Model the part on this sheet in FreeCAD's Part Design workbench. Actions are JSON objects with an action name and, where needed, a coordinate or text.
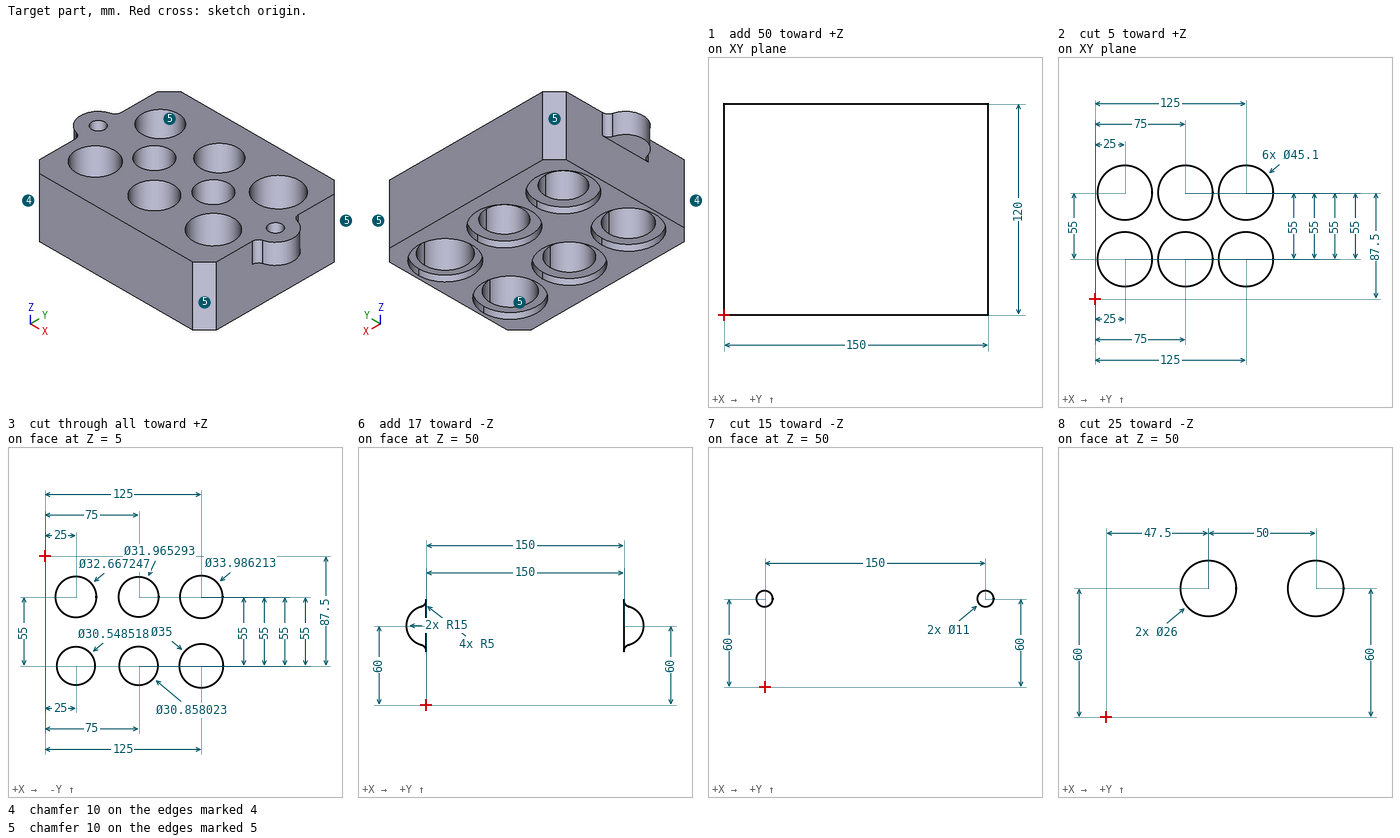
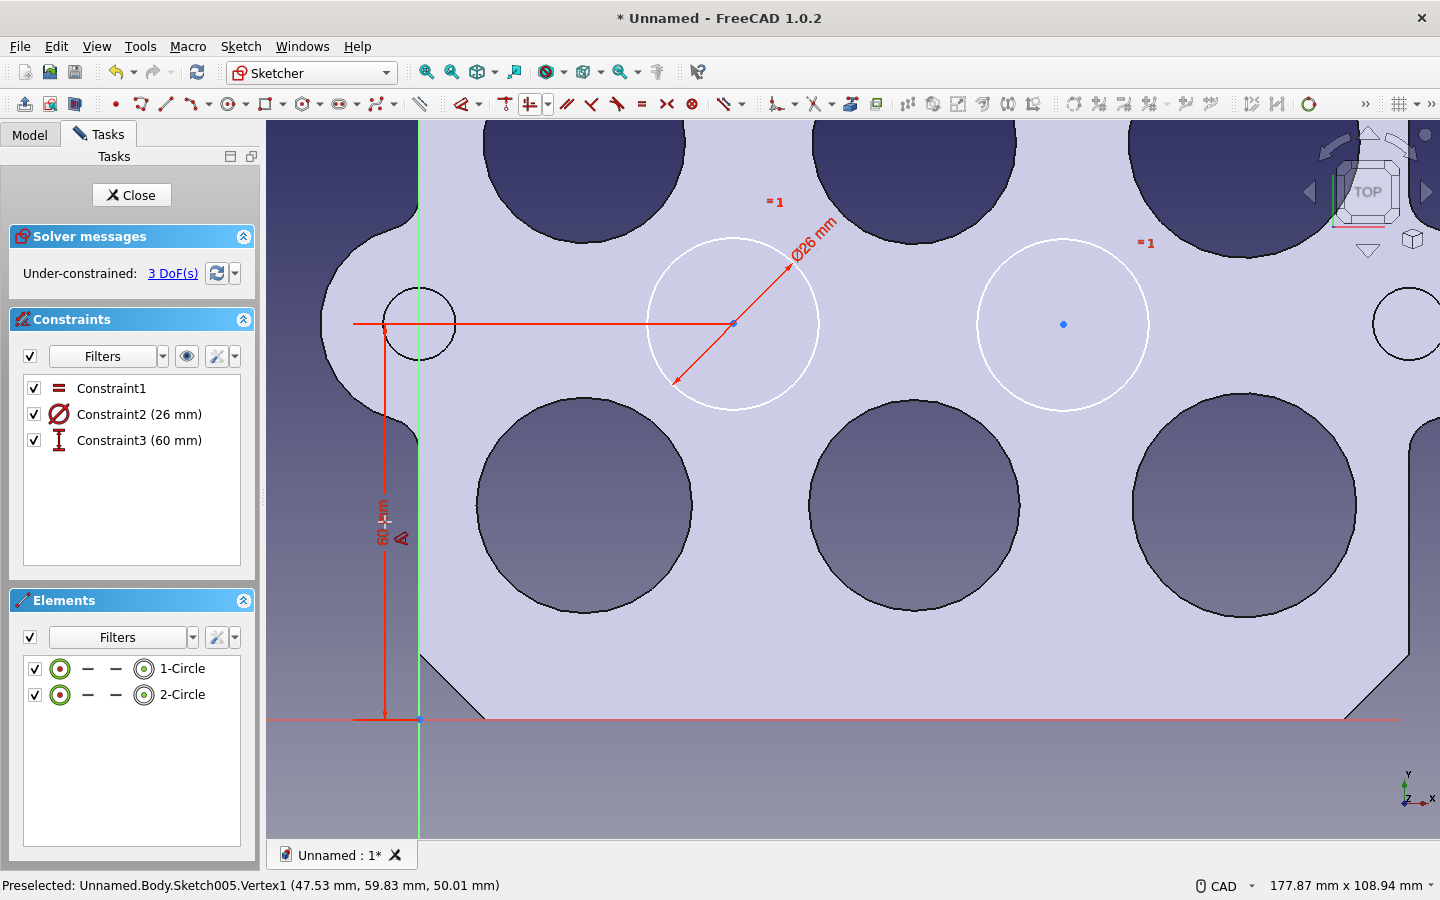
{"action": "left_click", "coordinate": [1063, 325]}
{"action": "left_click", "coordinate": [385, 432]}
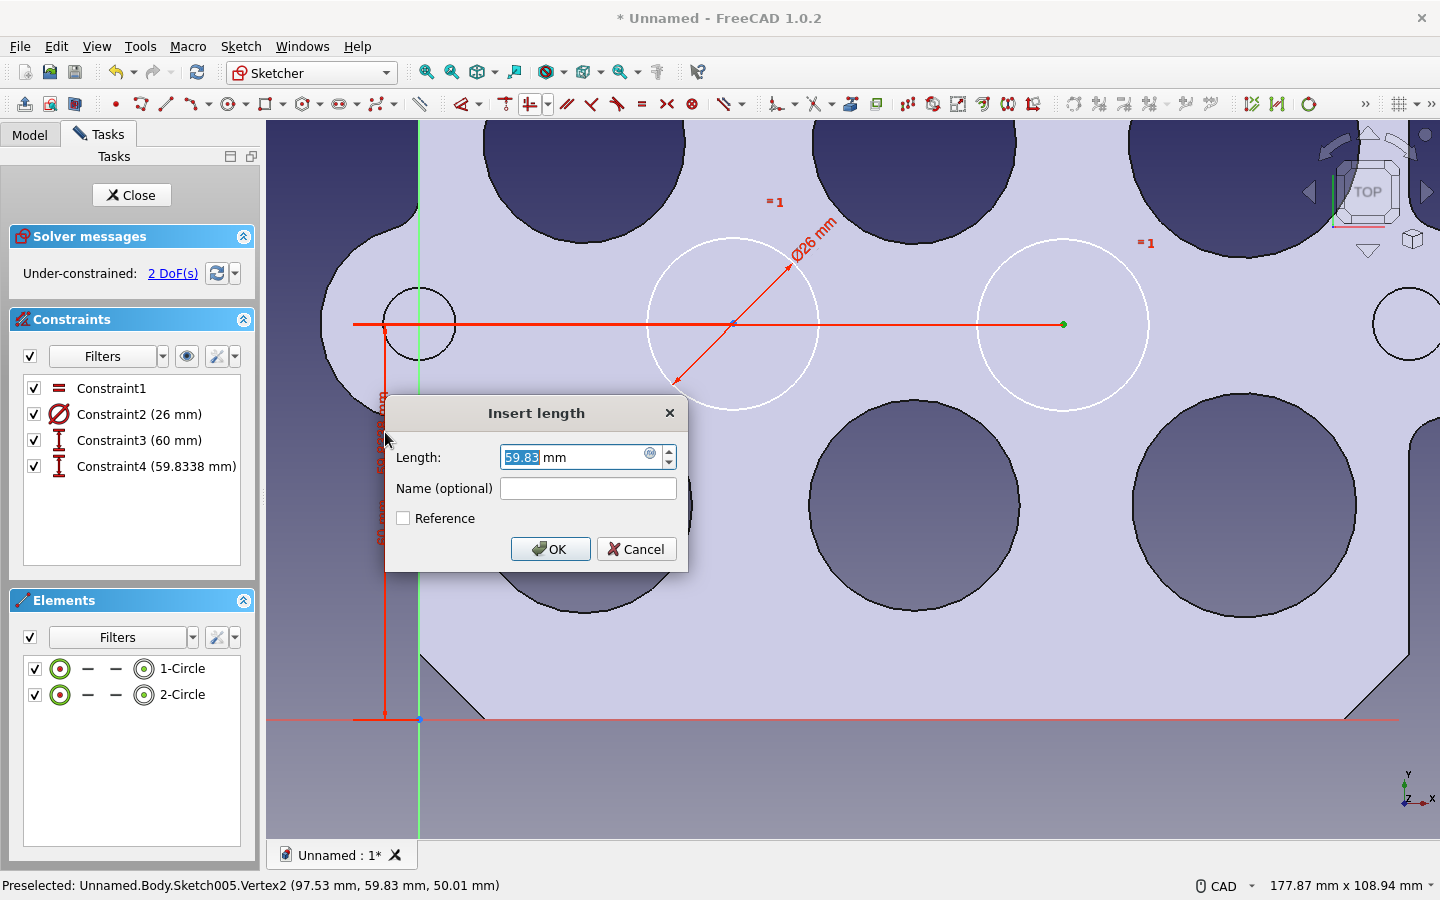
{"action": "type", "text": "60"}
{"action": "key", "text": "Return"}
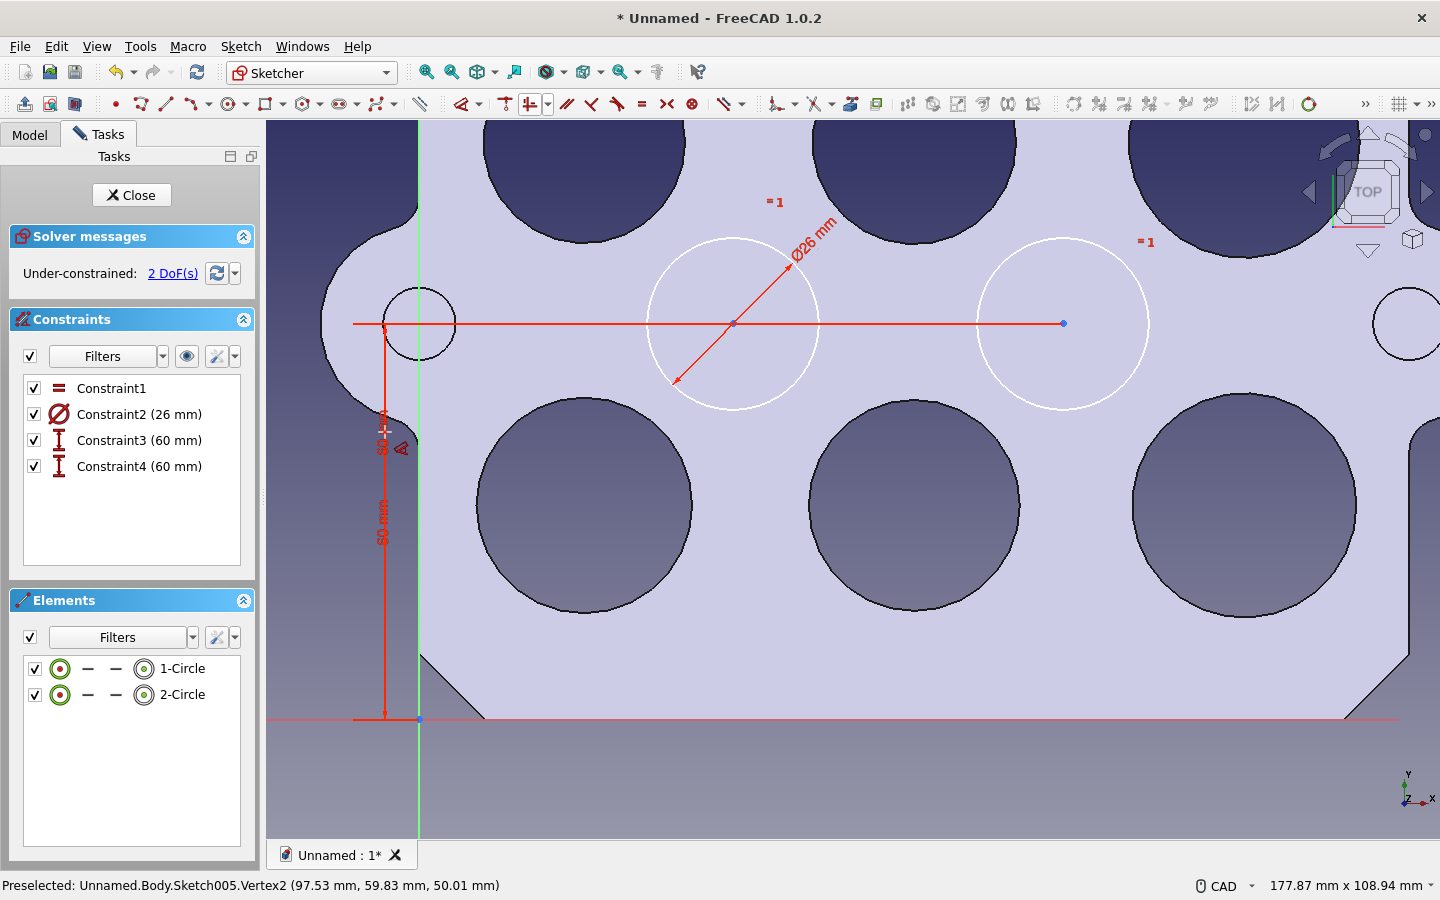
{"action": "left_click", "coordinate": [733, 324]}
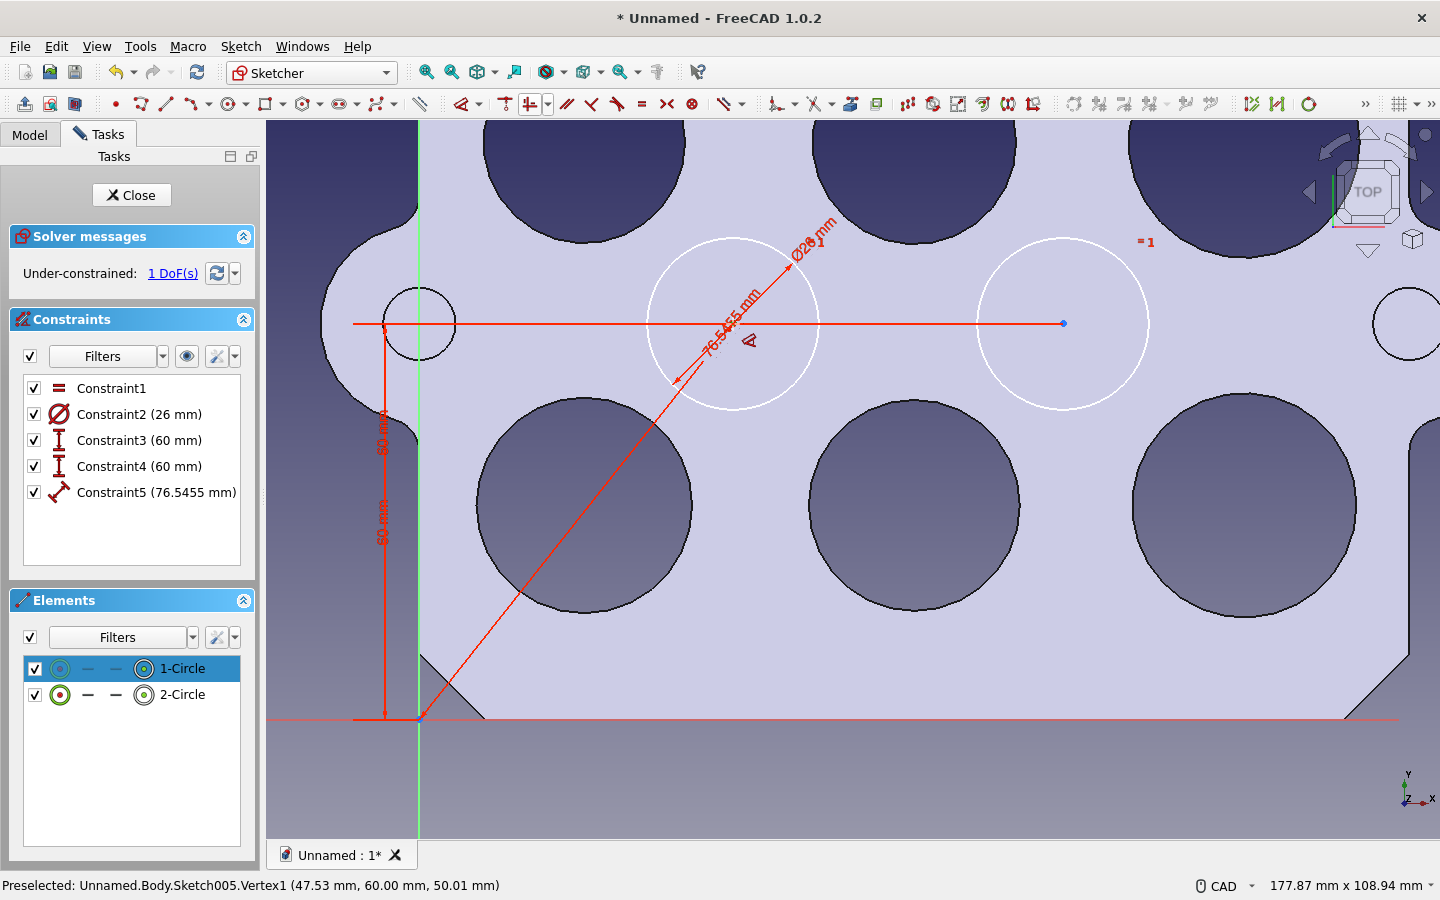
{"action": "left_click", "coordinate": [1063, 324]}
{"action": "left_click", "coordinate": [898, 290]}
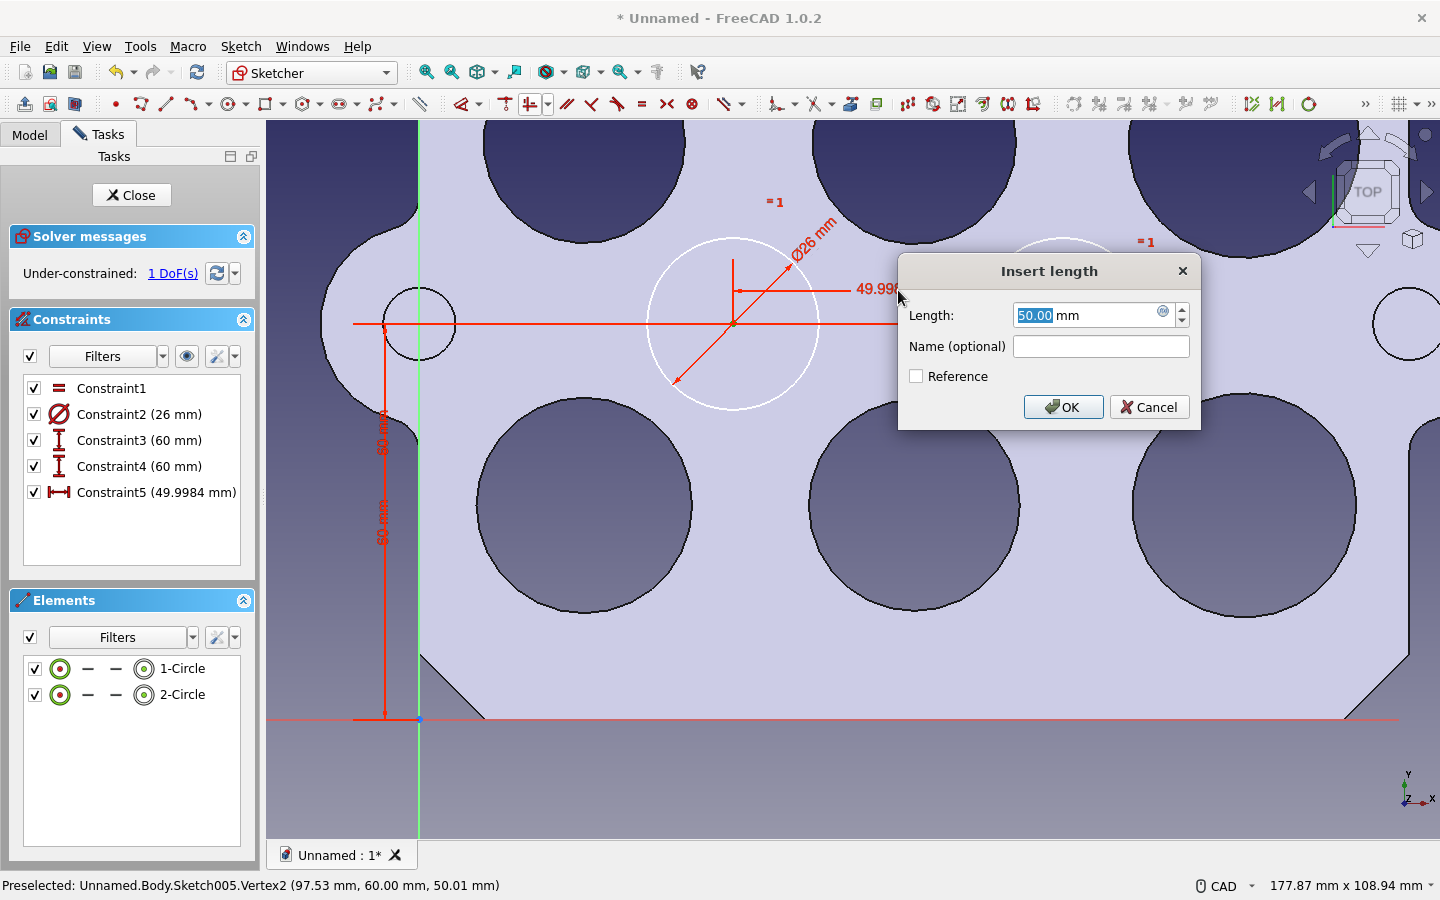
{"action": "type", "text": "50"}
{"action": "key", "text": "Return"}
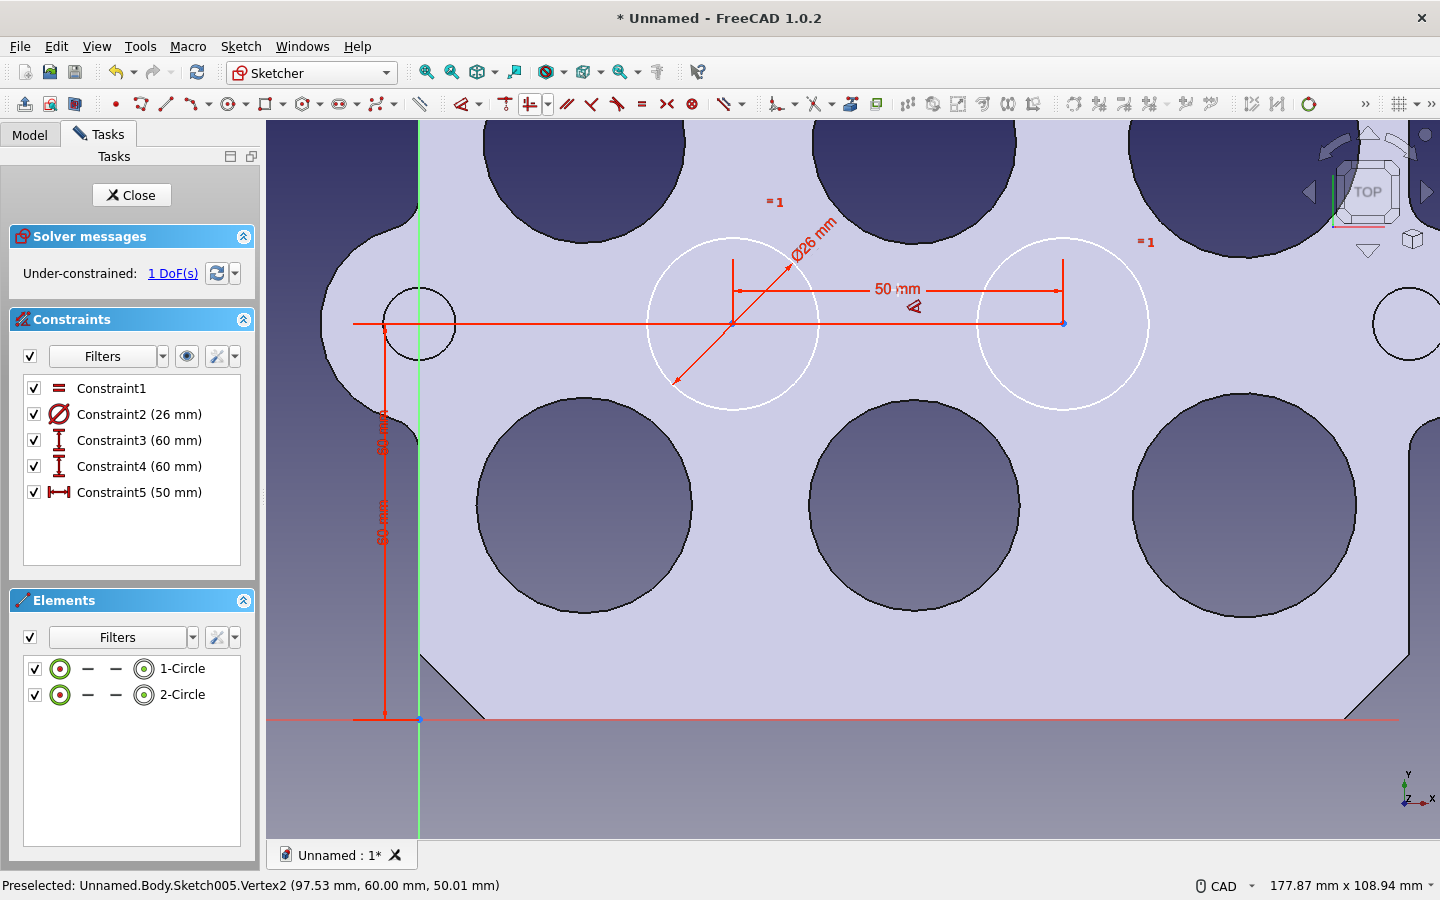
{"action": "left_click", "coordinate": [733, 324]}
{"action": "left_click", "coordinate": [576, 754]}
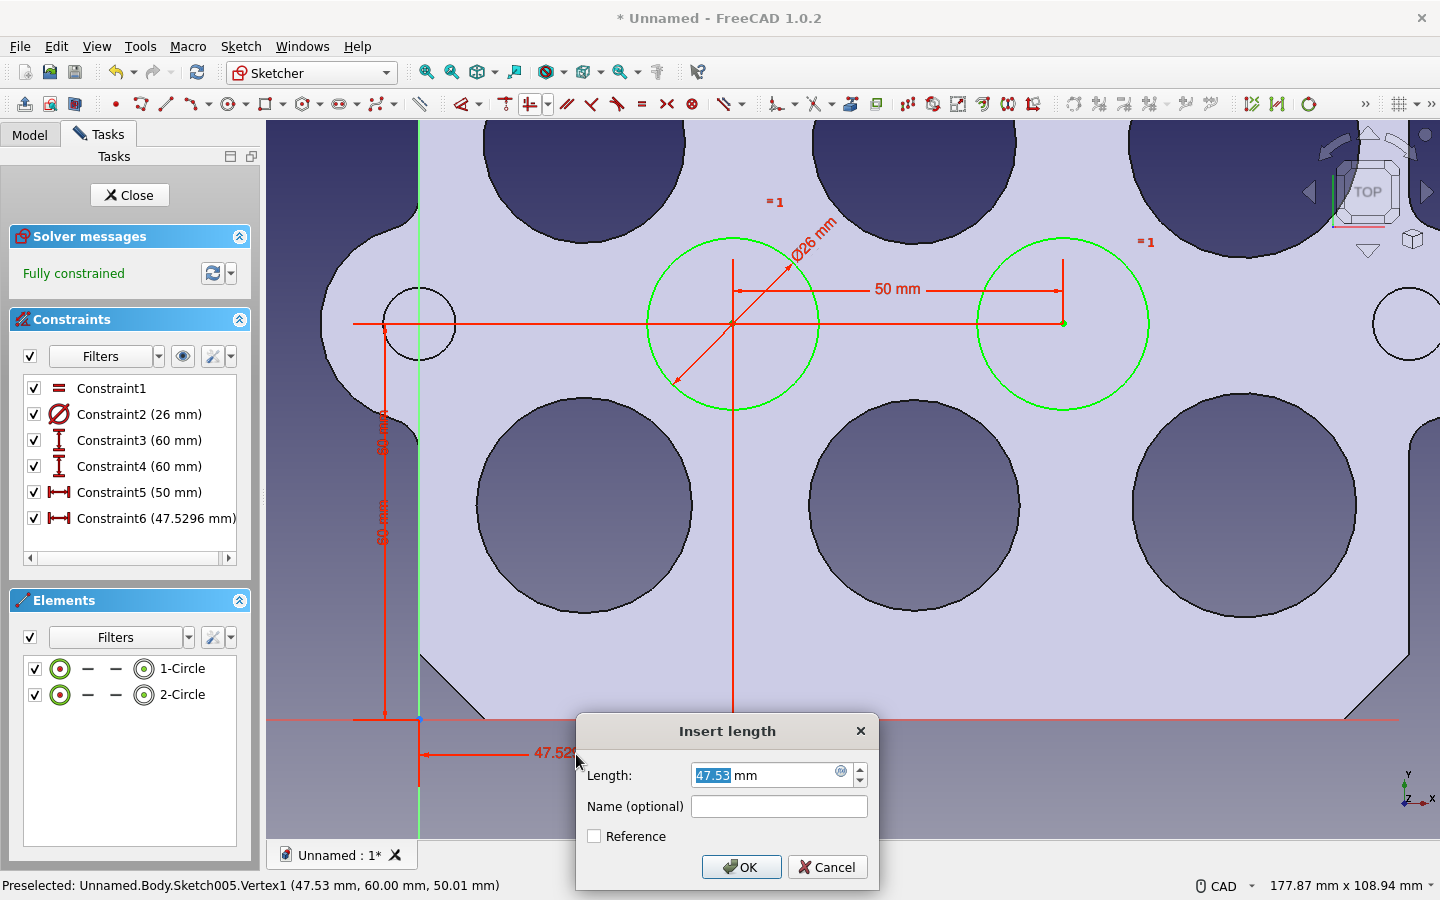
{"action": "type", "text": "47.5"}
{"action": "key", "text": "Return"}
{"action": "key", "text": "Escape"}